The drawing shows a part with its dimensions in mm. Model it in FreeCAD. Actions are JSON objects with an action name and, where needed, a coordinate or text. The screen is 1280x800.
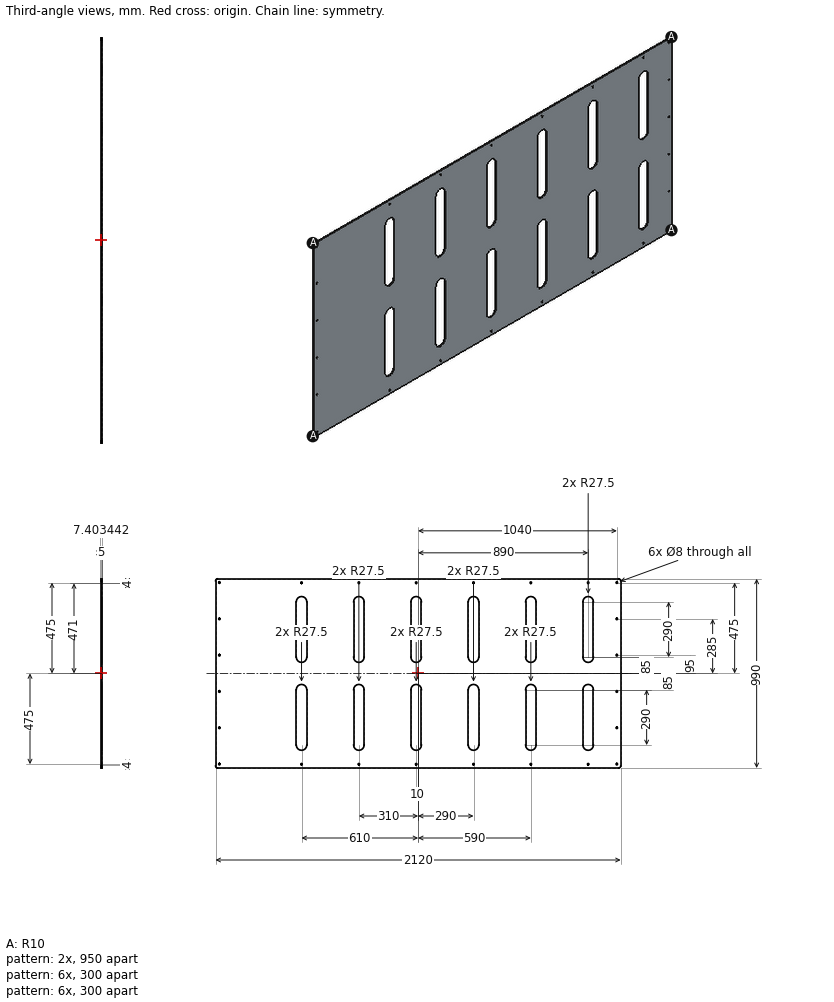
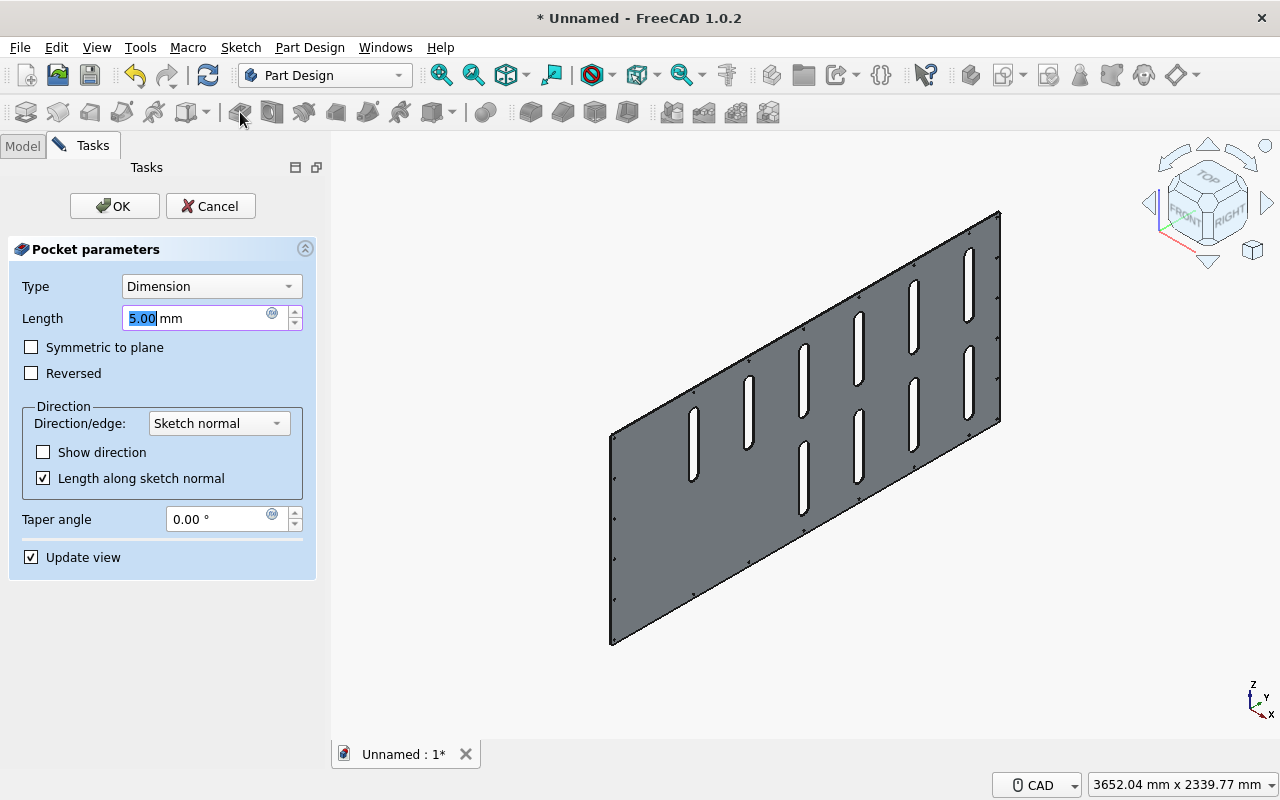
{"action": "type", "text": "10"}
{"action": "key", "text": "Tab"}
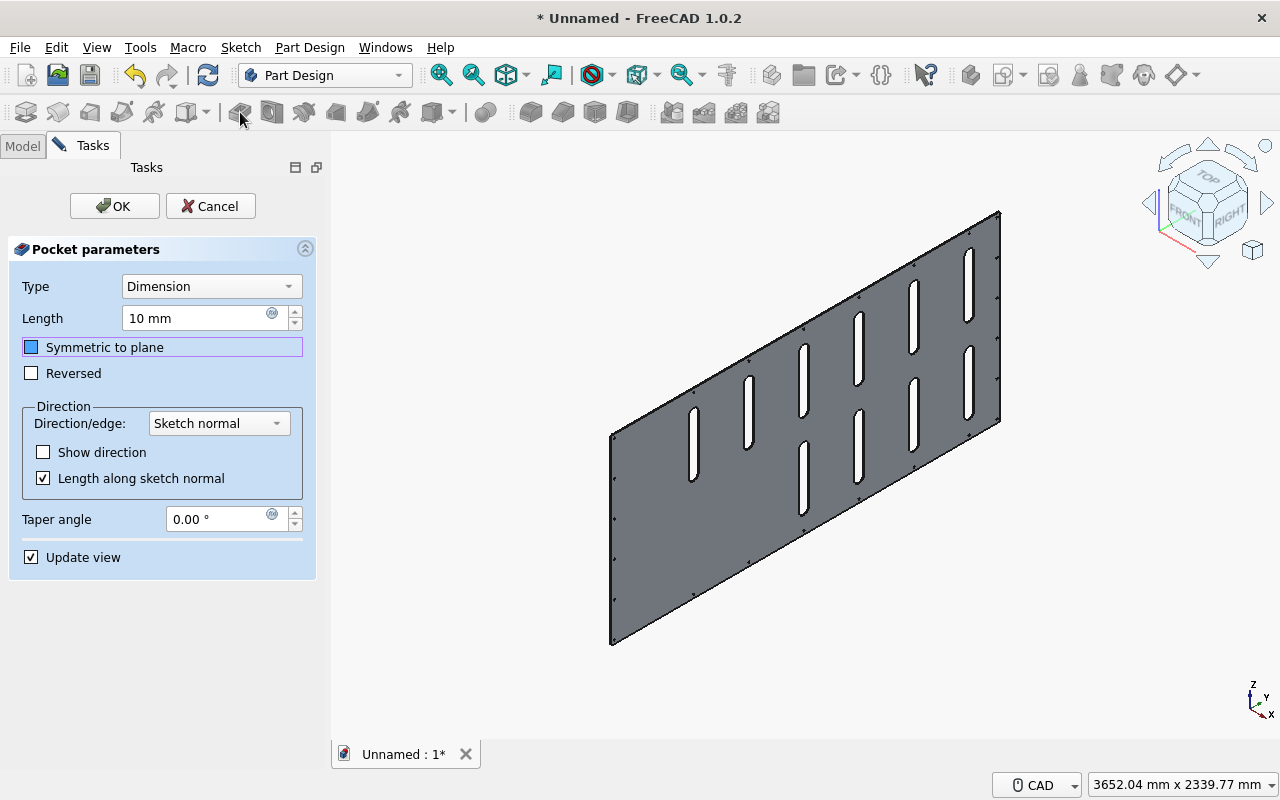
{"action": "left_click", "coordinate": [115, 206]}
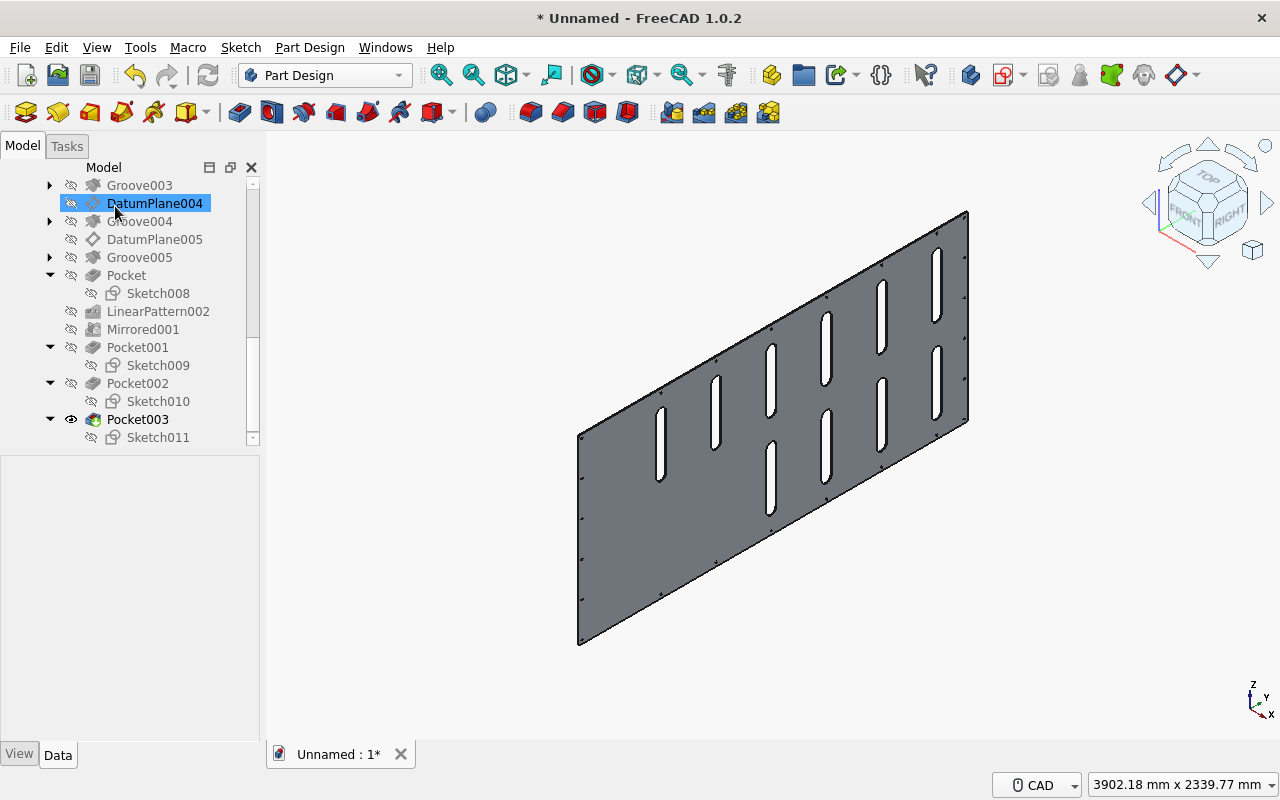
{"action": "left_click", "coordinate": [718, 490]}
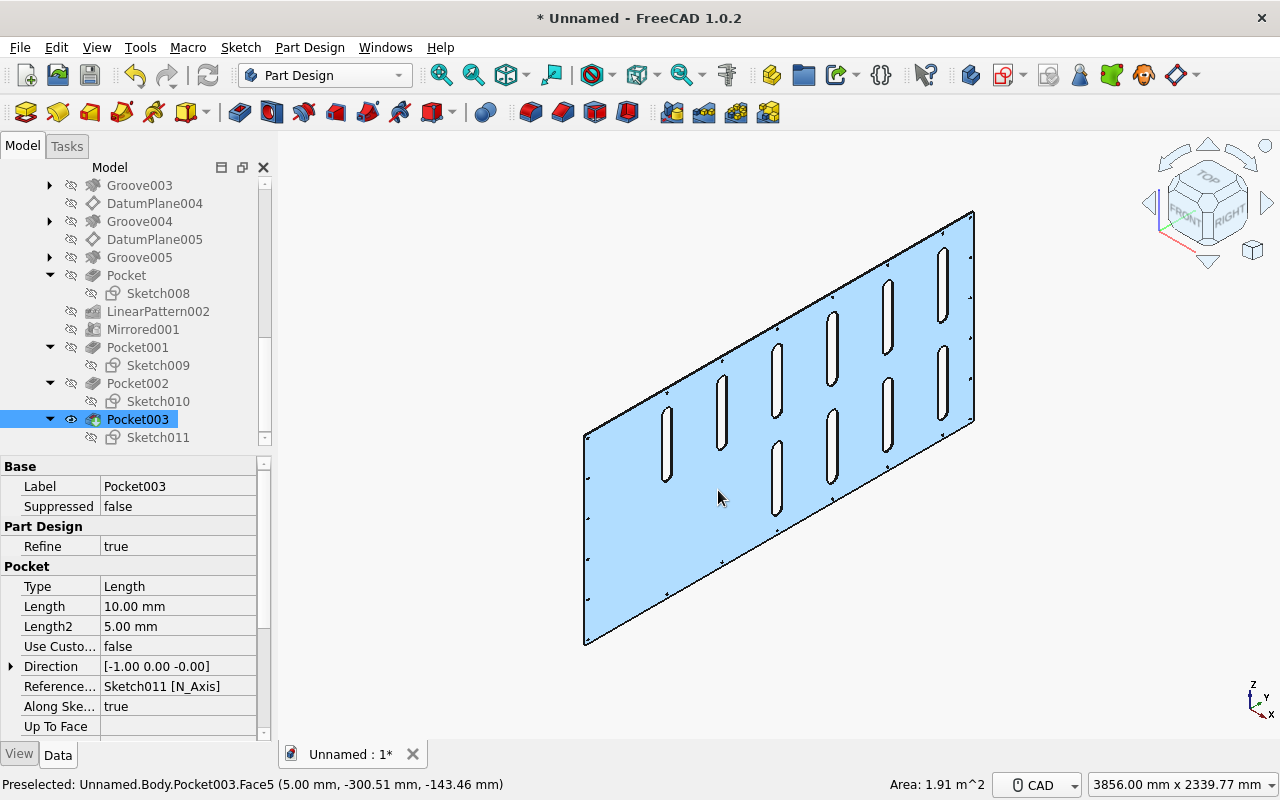
{"action": "left_click", "coordinate": [1004, 76]}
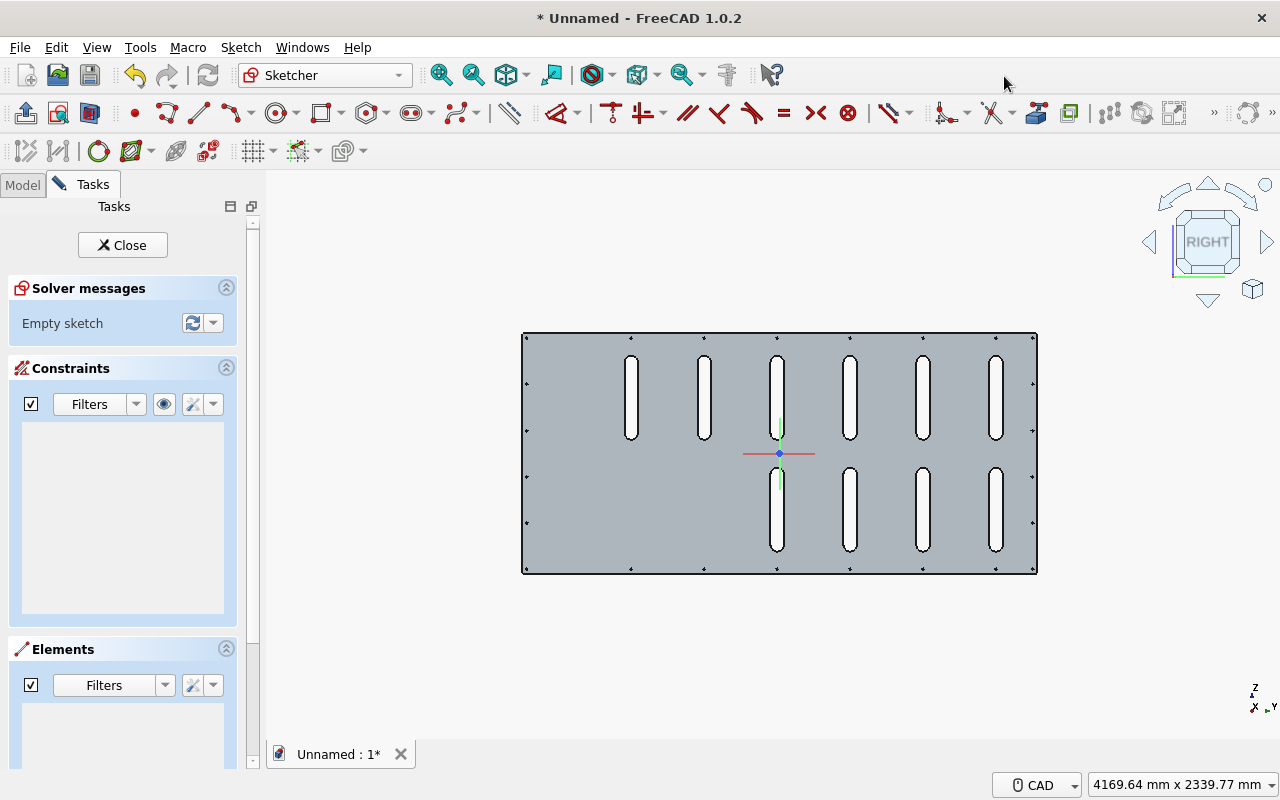
{"action": "scroll", "coordinate": [750, 518], "scroll_direction": "up", "scroll_amount": 7}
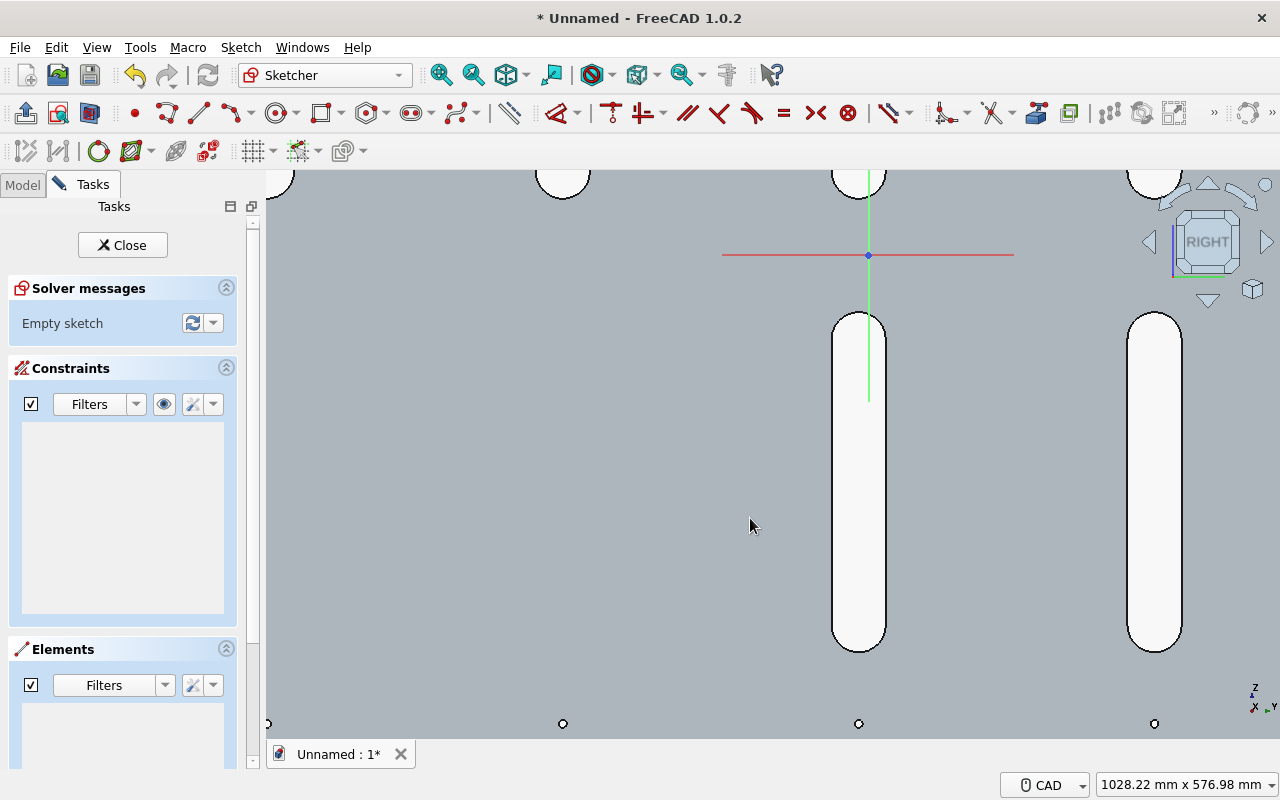
{"action": "left_click", "coordinate": [412, 114]}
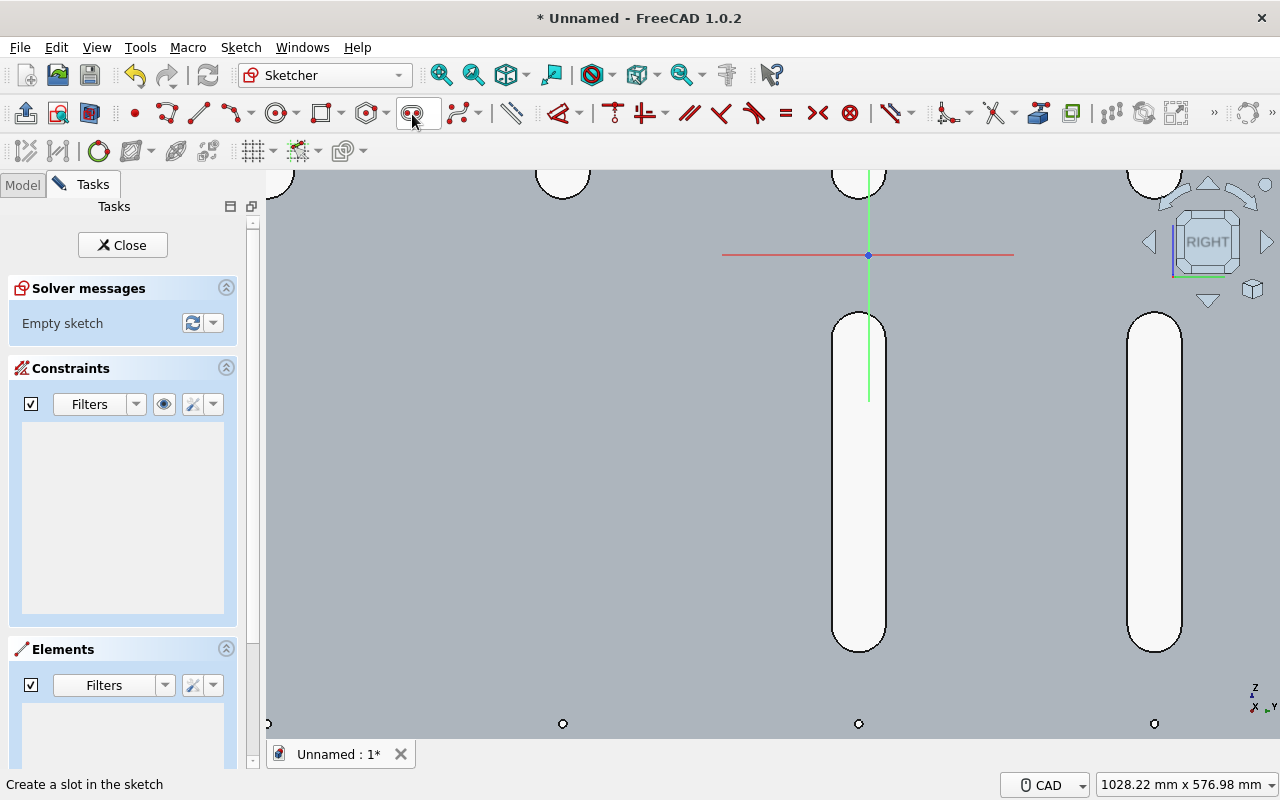
{"action": "left_click", "coordinate": [563, 625]}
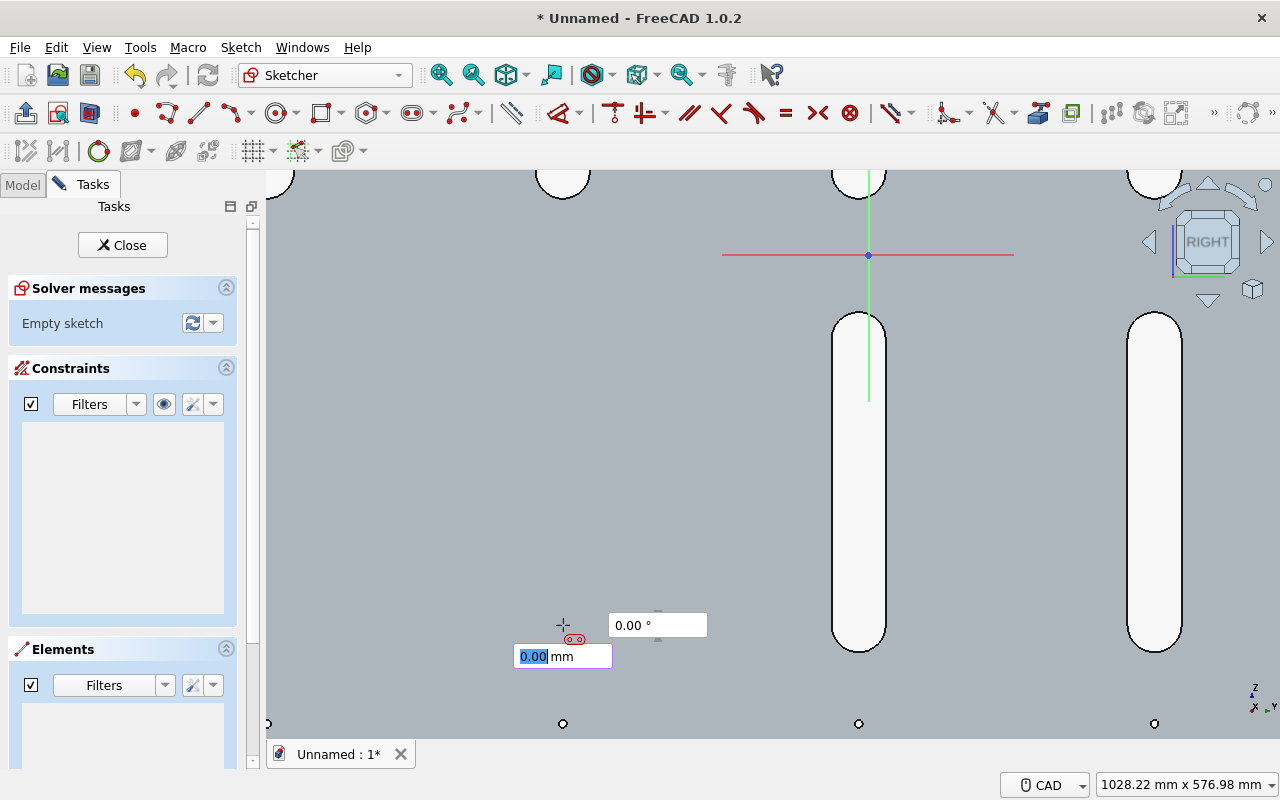
{"action": "left_click", "coordinate": [563, 339]}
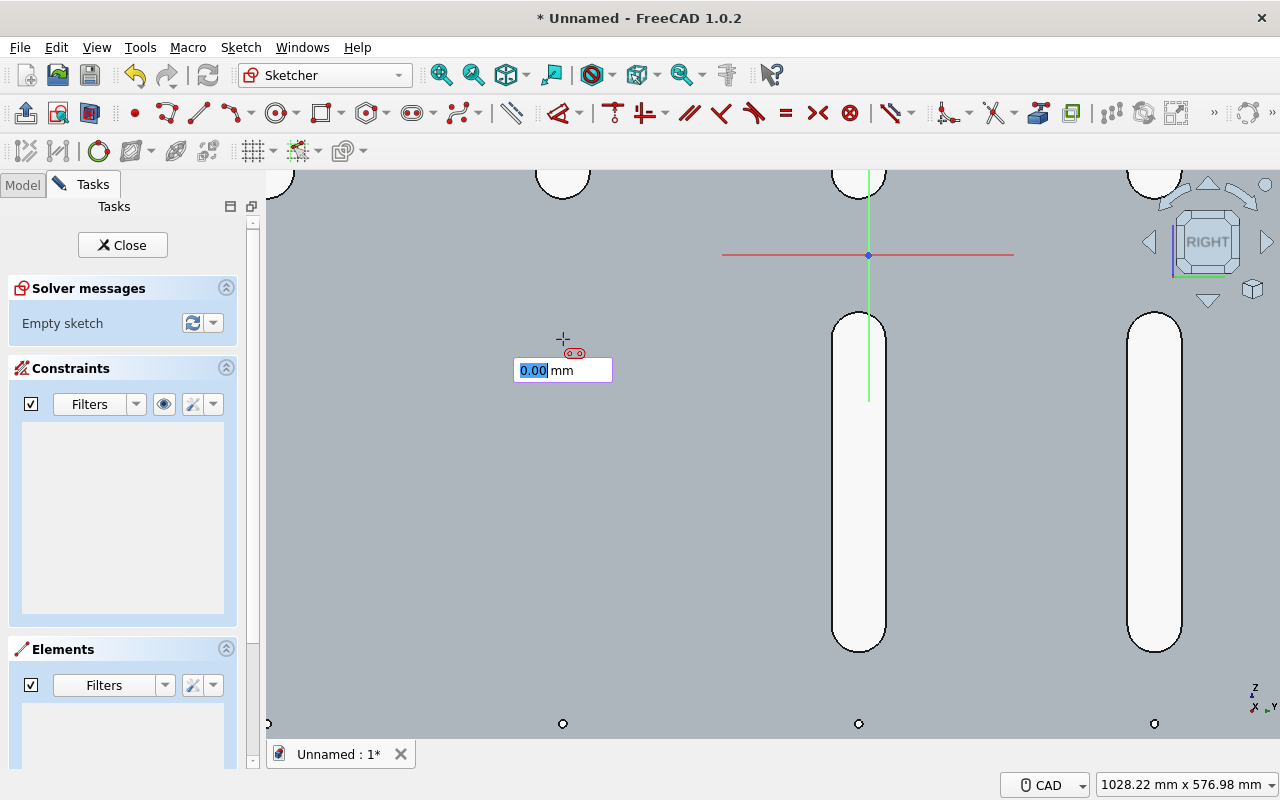
{"action": "left_click", "coordinate": [590, 482]}
{"action": "key", "text": "Escape"}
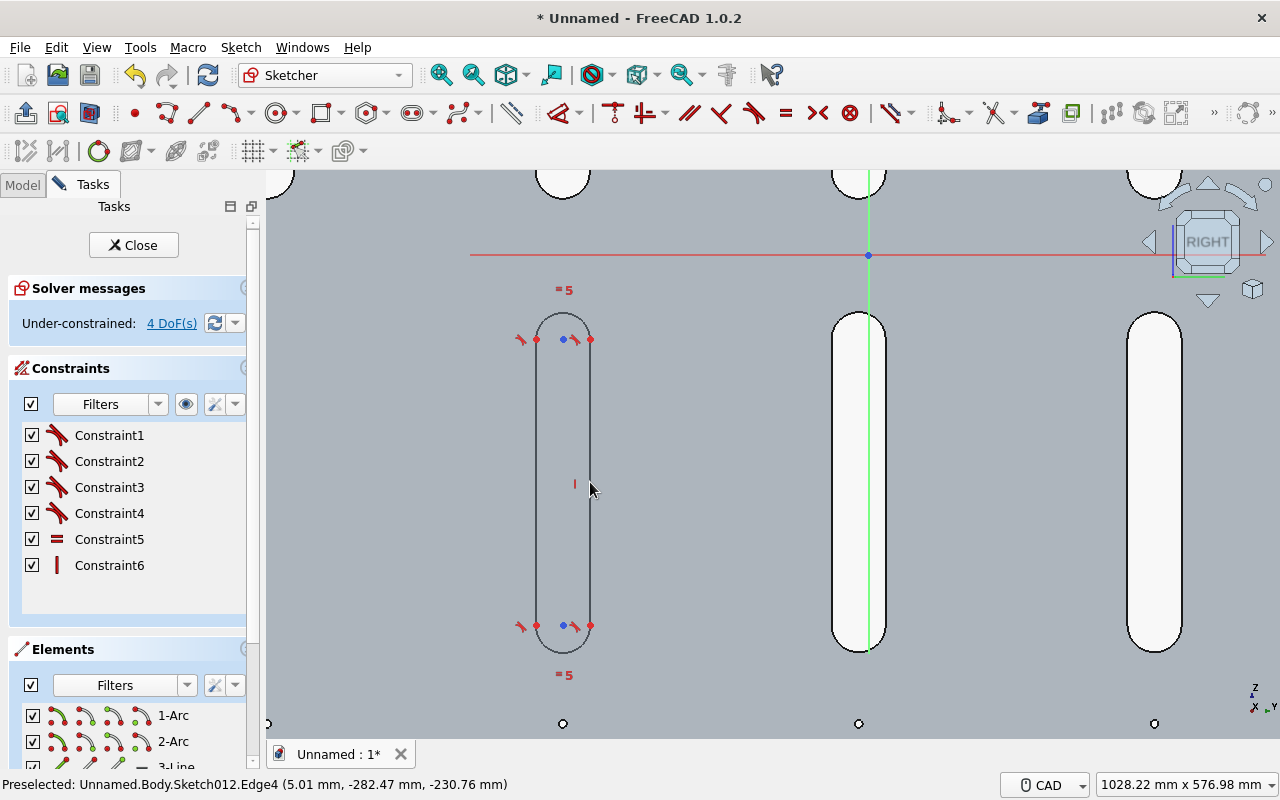
{"action": "key", "text": "d"}